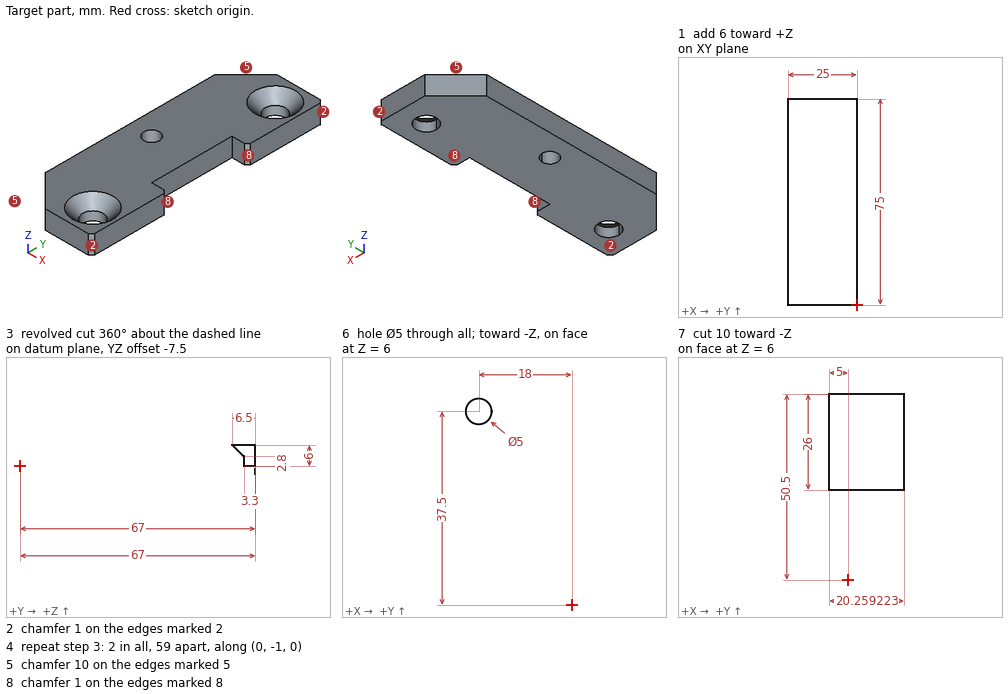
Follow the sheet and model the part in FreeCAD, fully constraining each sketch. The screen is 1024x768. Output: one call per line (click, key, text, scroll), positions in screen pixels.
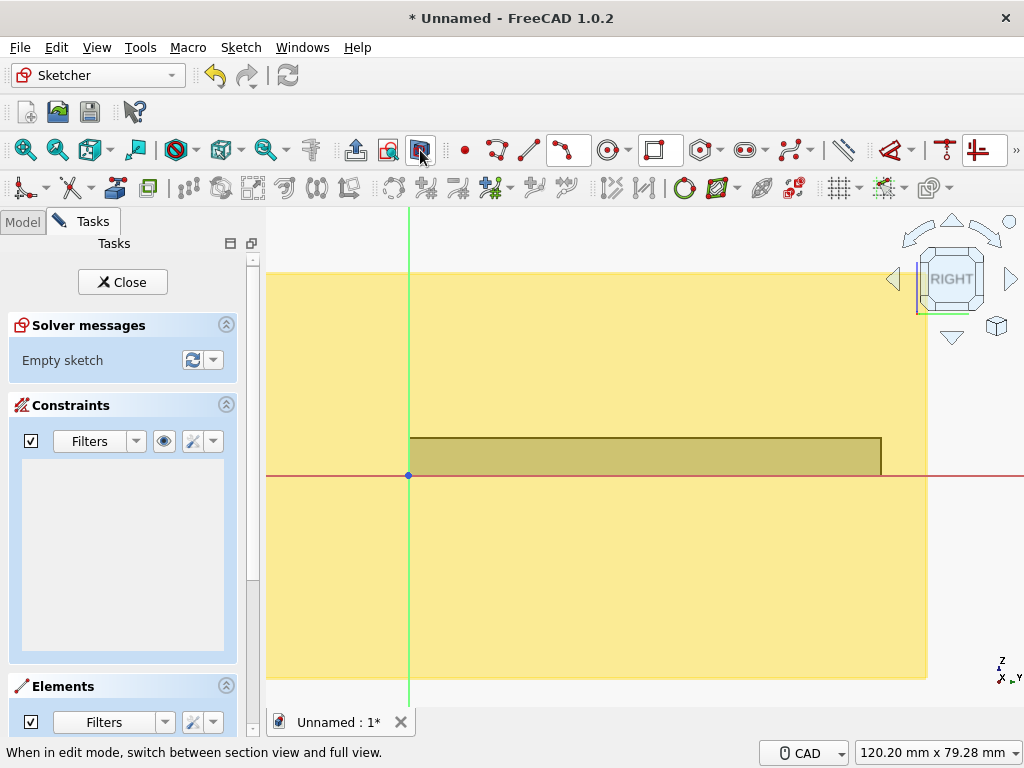
scroll(857, 466, up, 9)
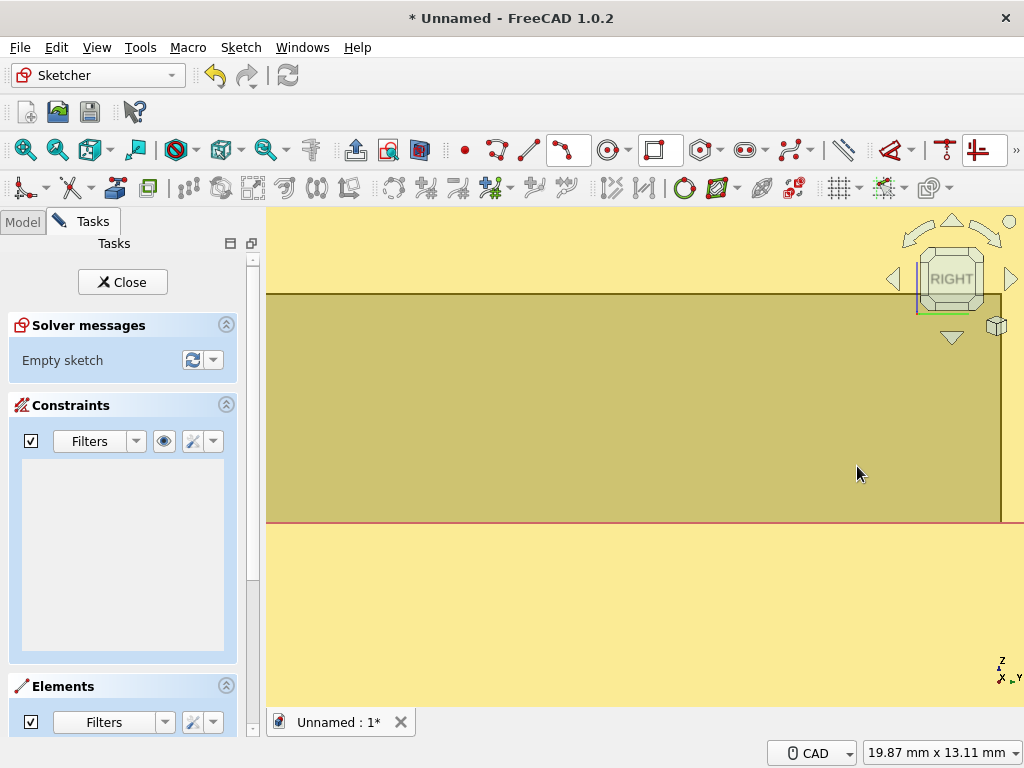
click(498, 150)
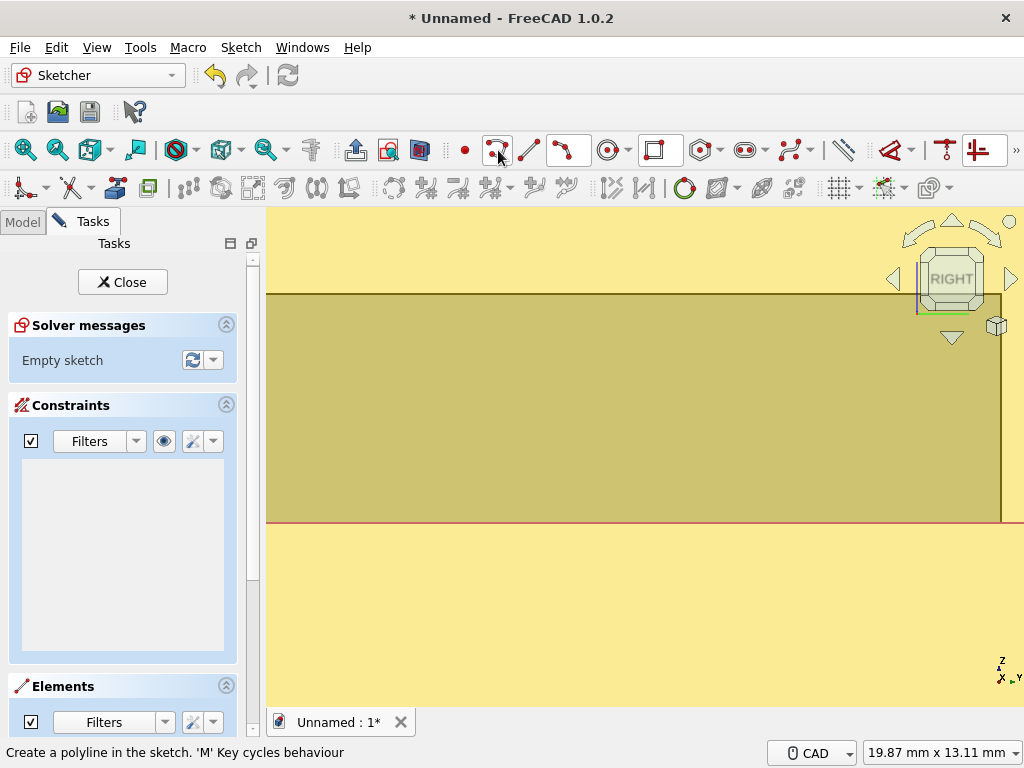
click(448, 294)
click(570, 417)
click(570, 523)
click(696, 514)
click(696, 294)
click(448, 295)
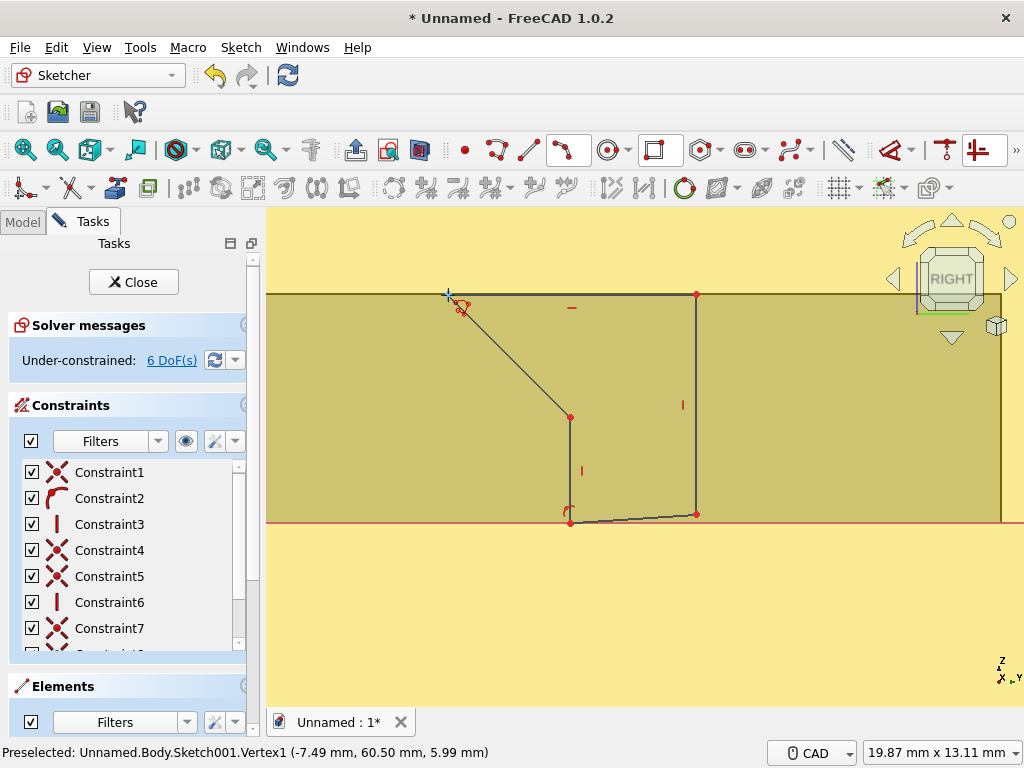
click(530, 150)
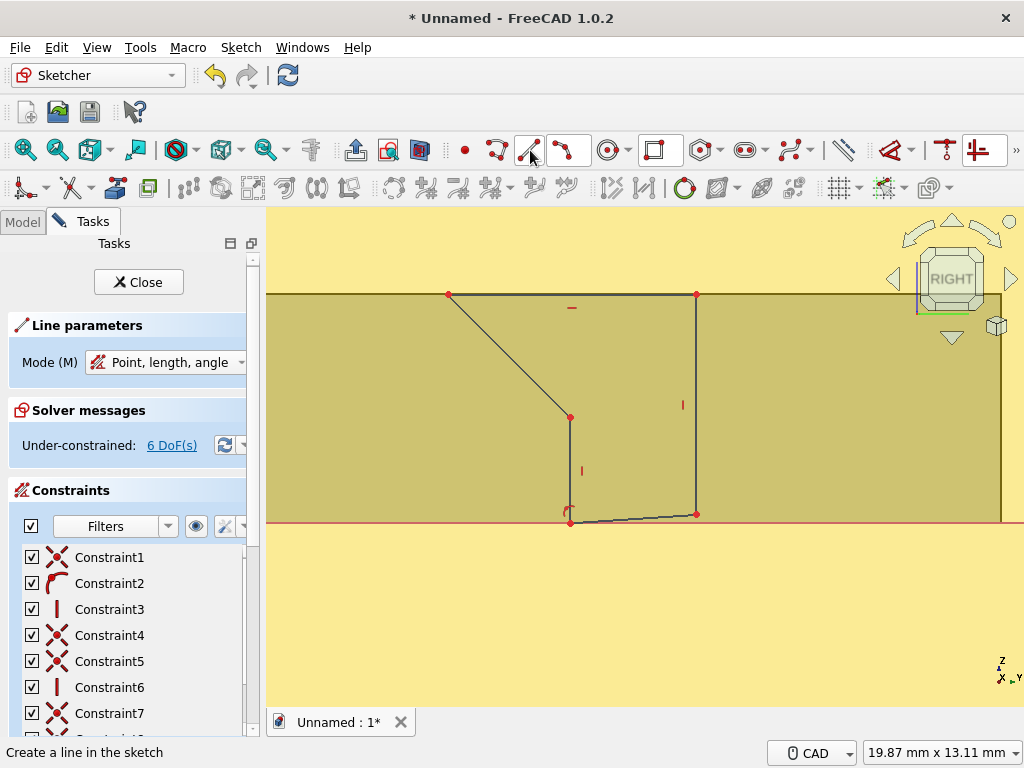
click(696, 546)
click(696, 615)
key(Escape)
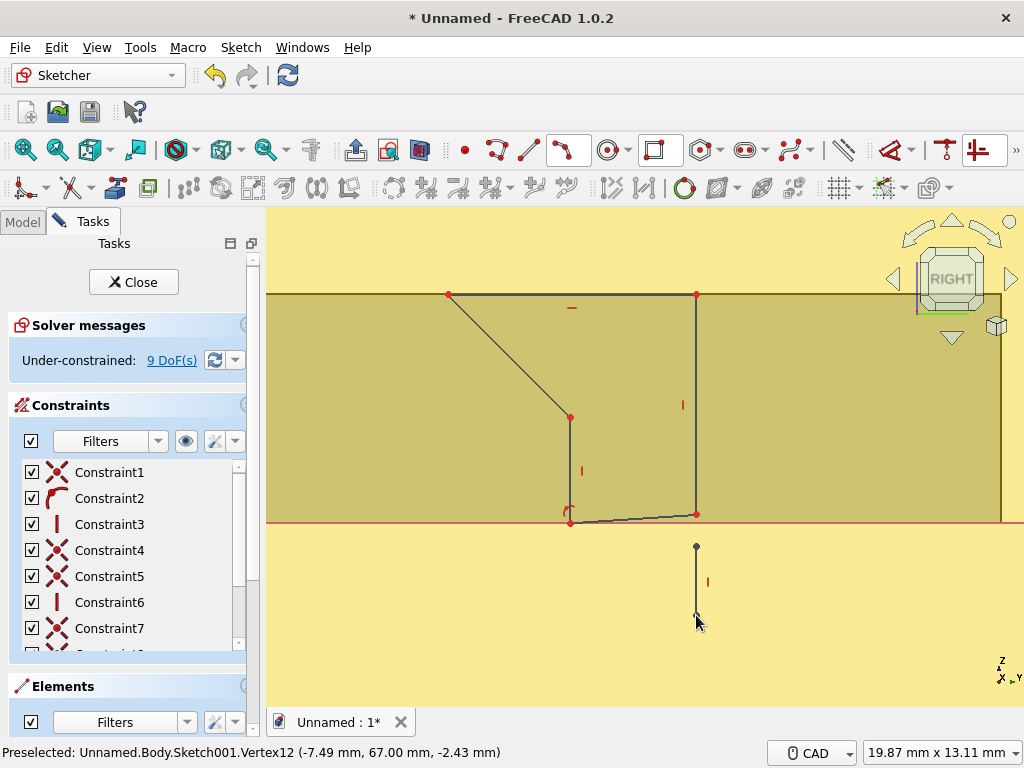
click(696, 568)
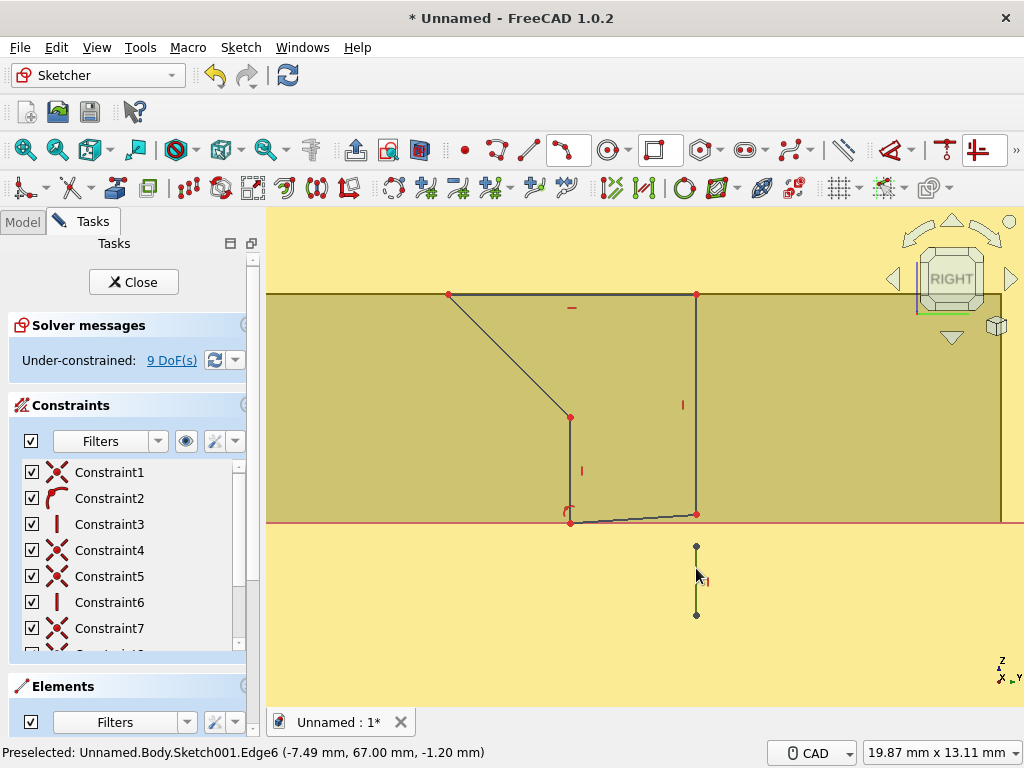
click(844, 150)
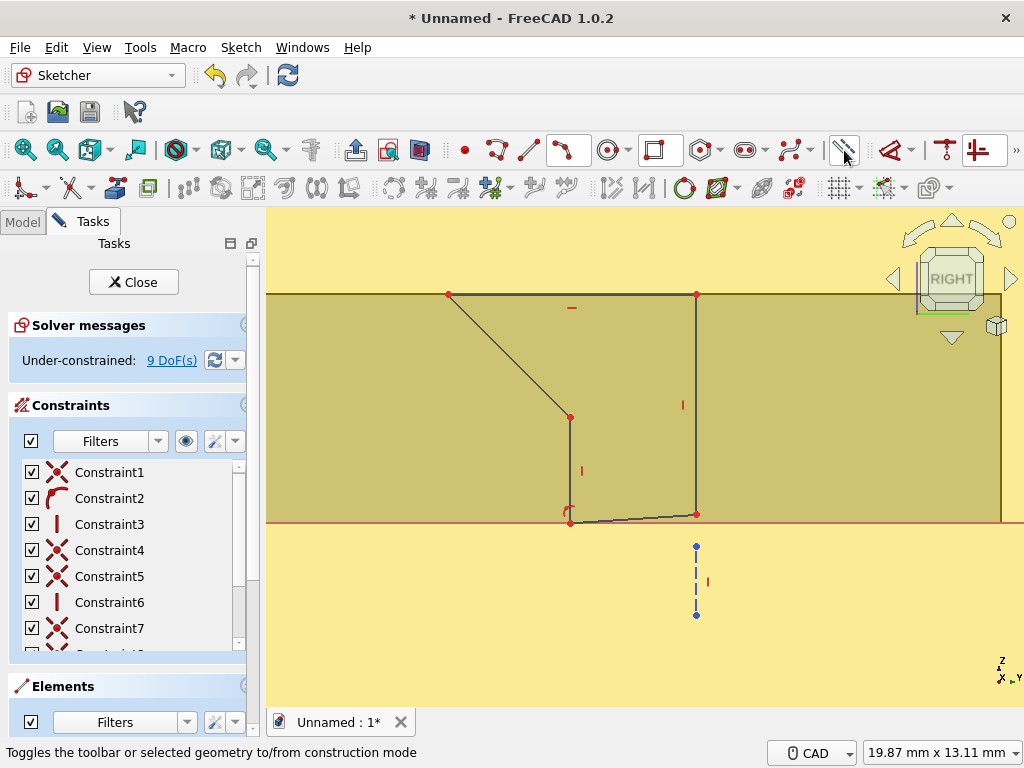
click(608, 521)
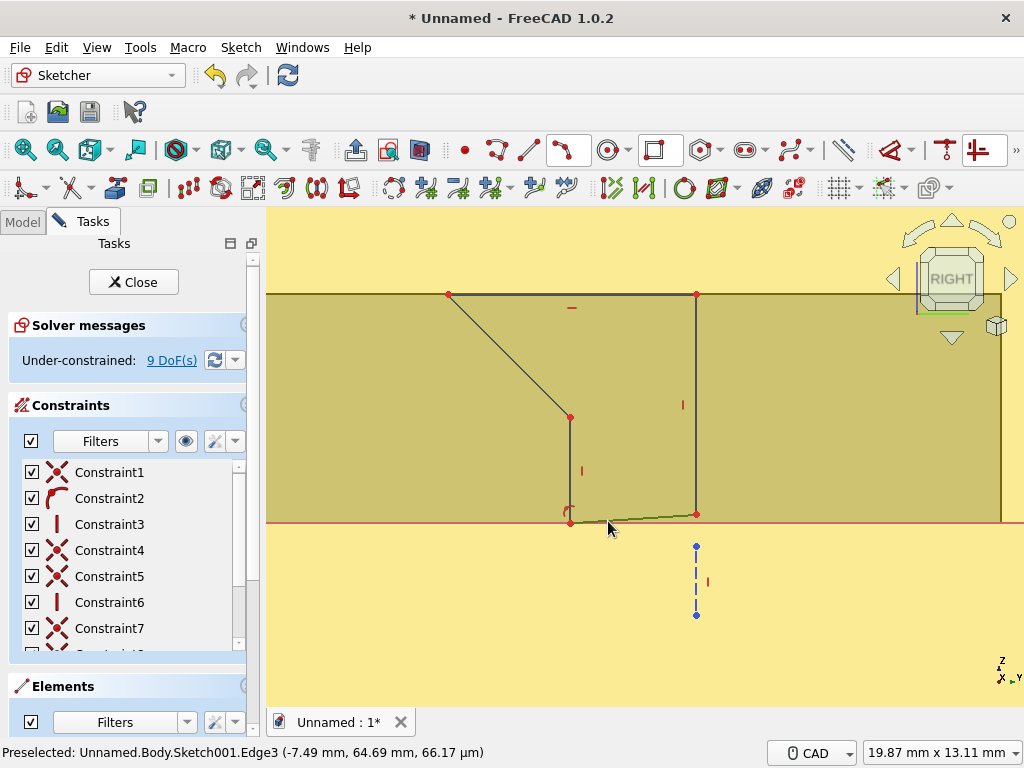
key(h)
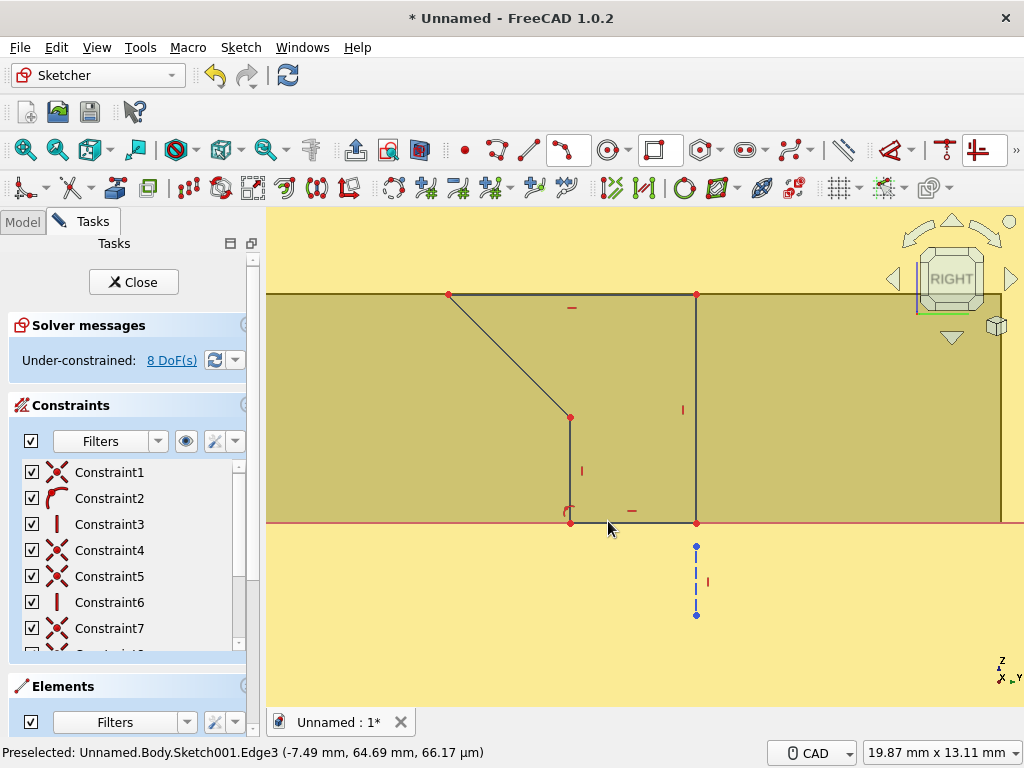
click(890, 150)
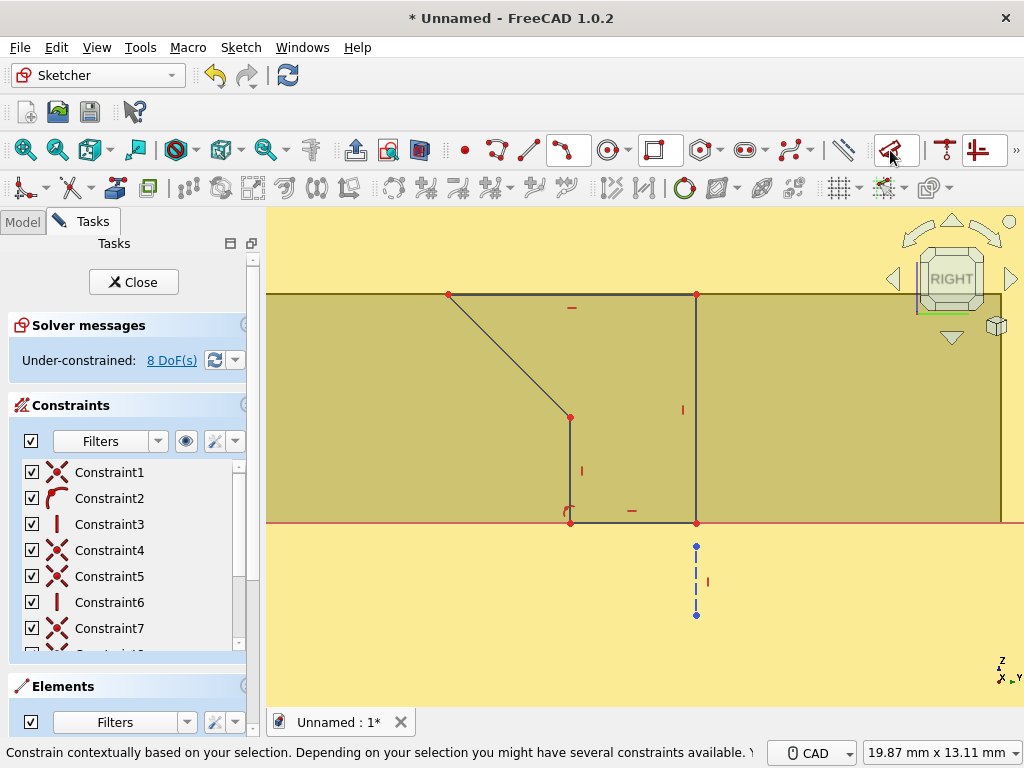
click(696, 455)
click(730, 409)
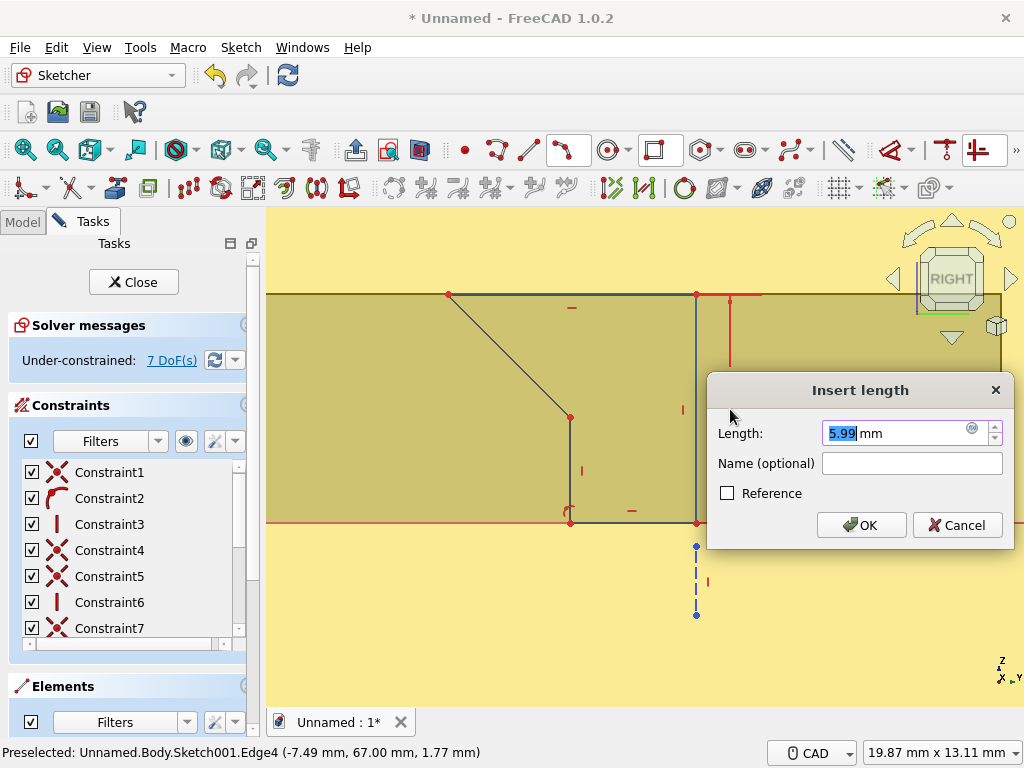
text(6)
key(Return)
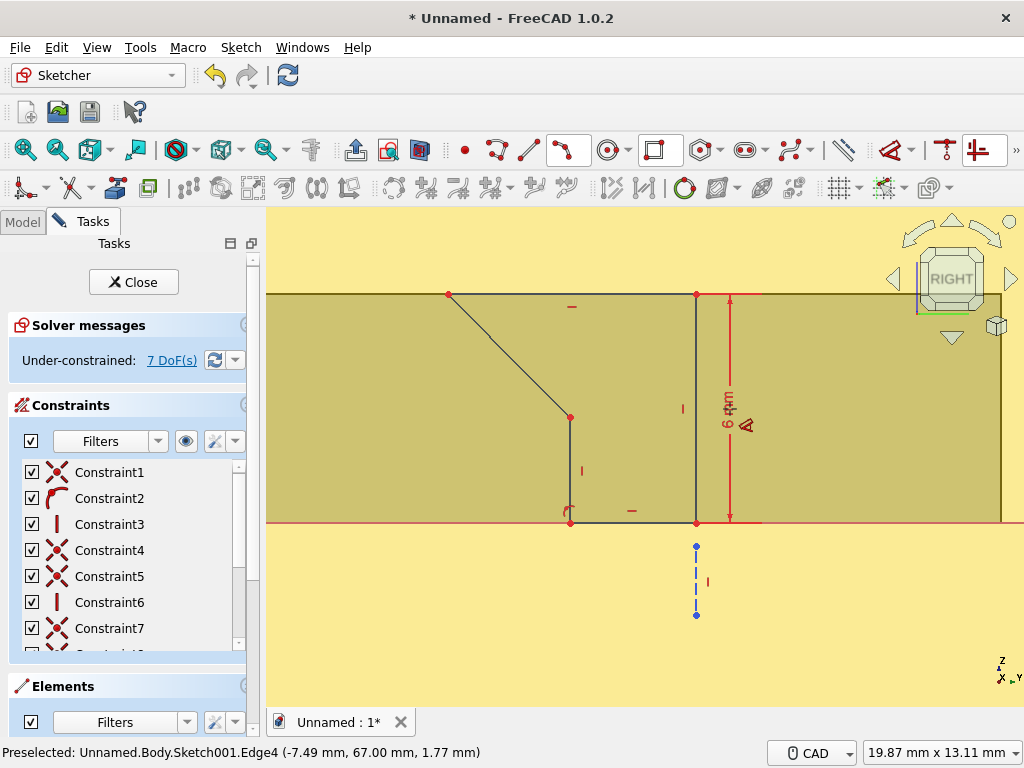
click(570, 450)
click(536, 471)